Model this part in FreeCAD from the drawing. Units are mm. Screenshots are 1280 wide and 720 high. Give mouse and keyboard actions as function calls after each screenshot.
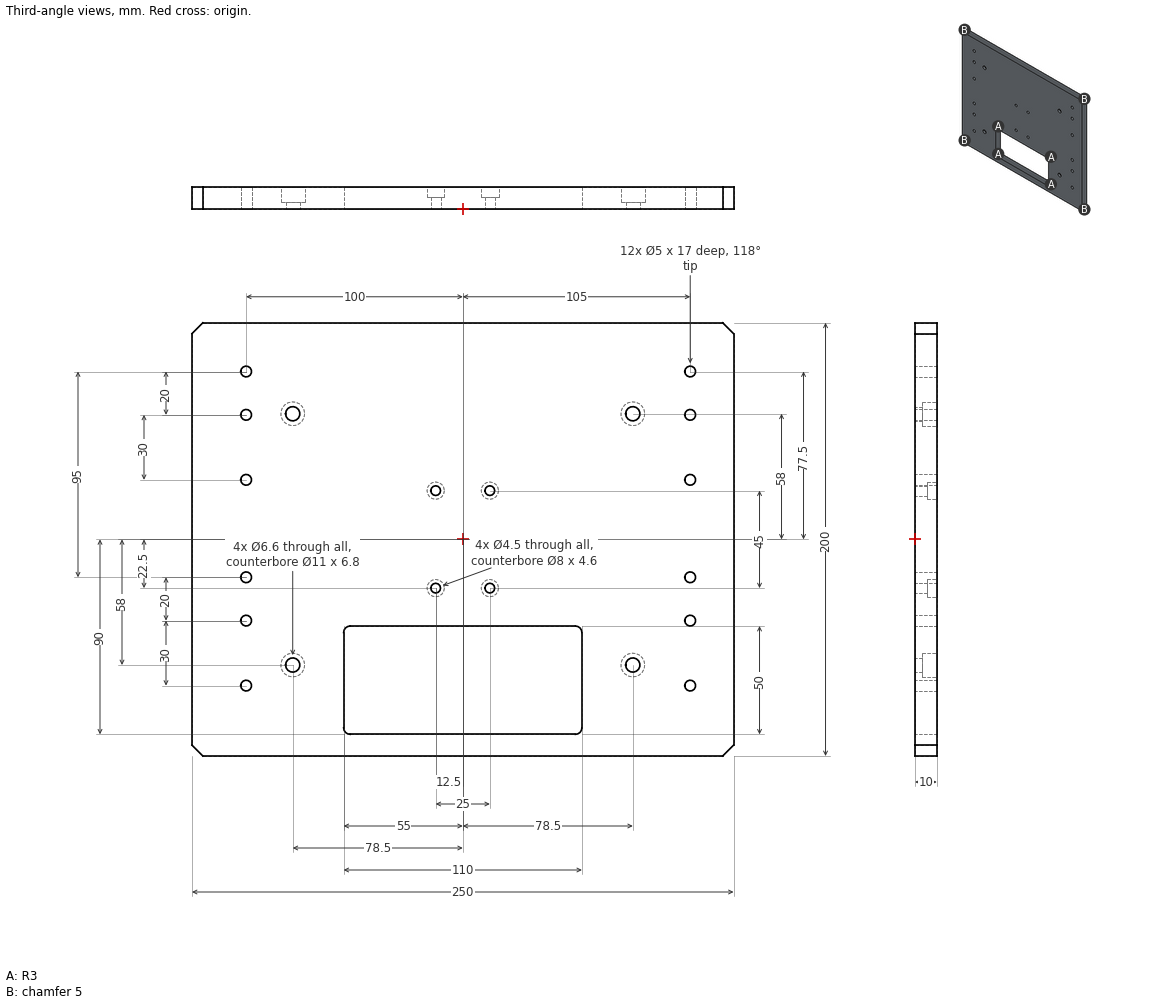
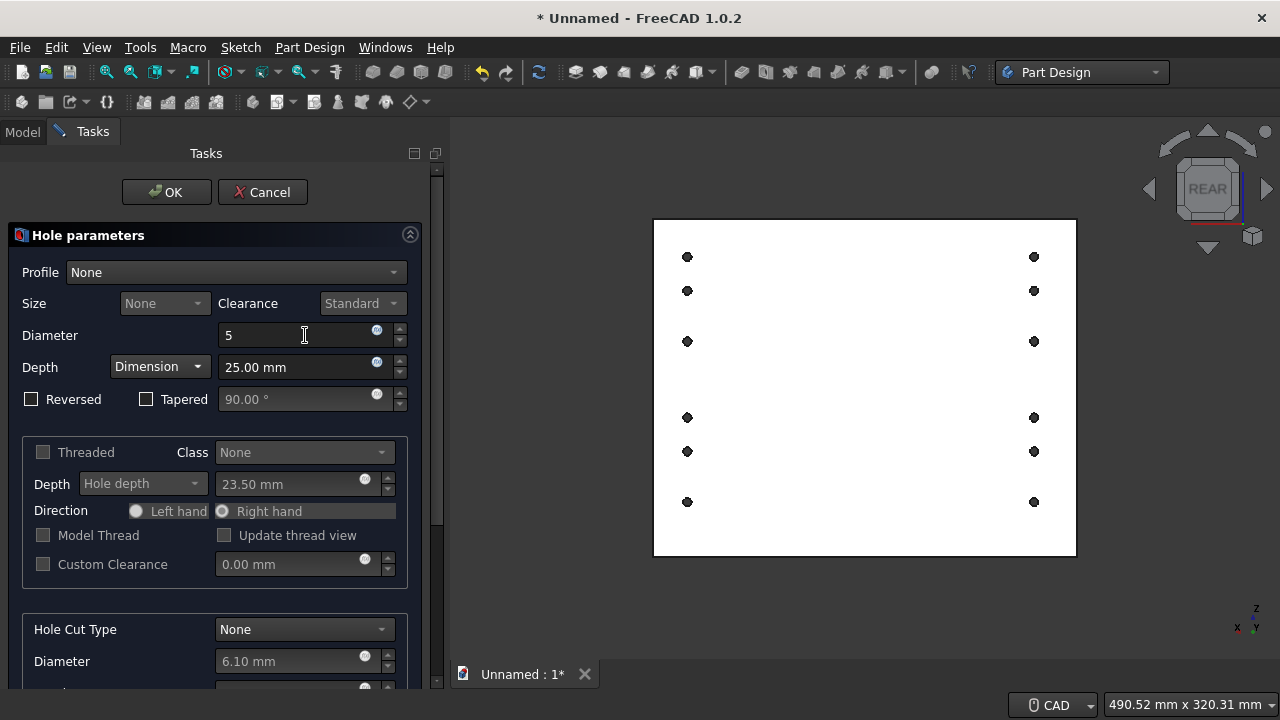
triple_click(305, 367)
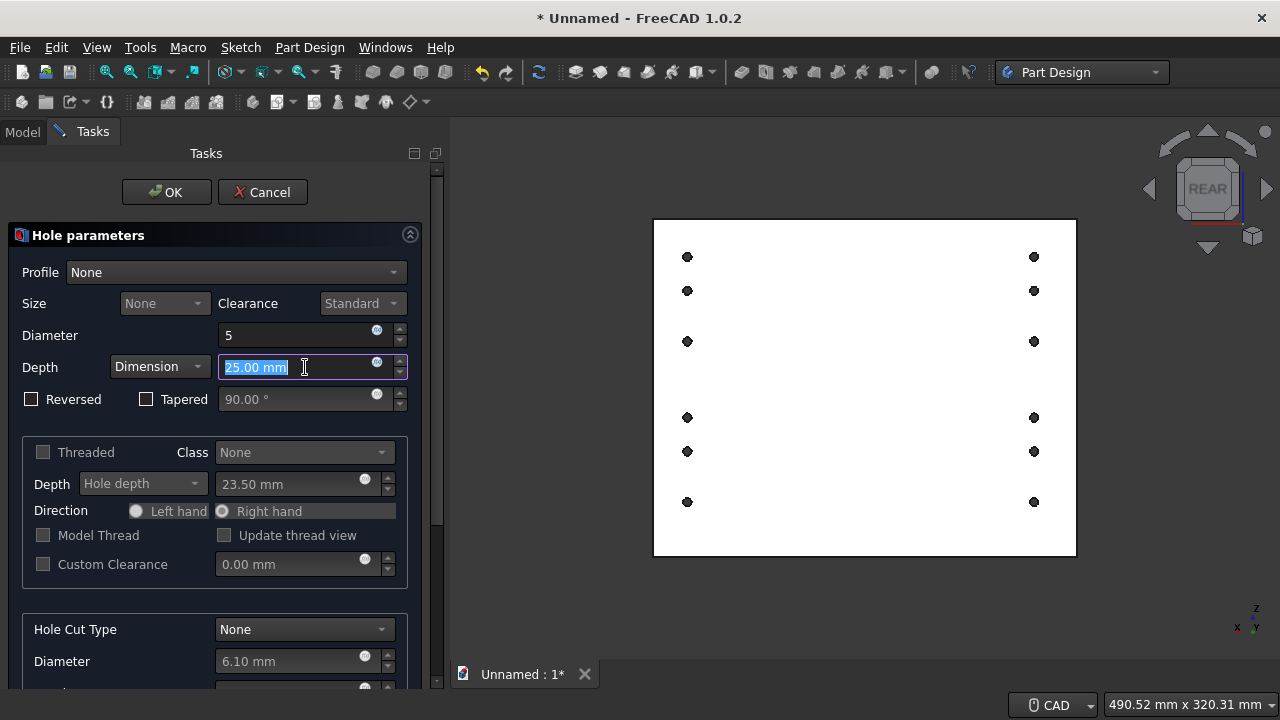
text(17)
key(Tab)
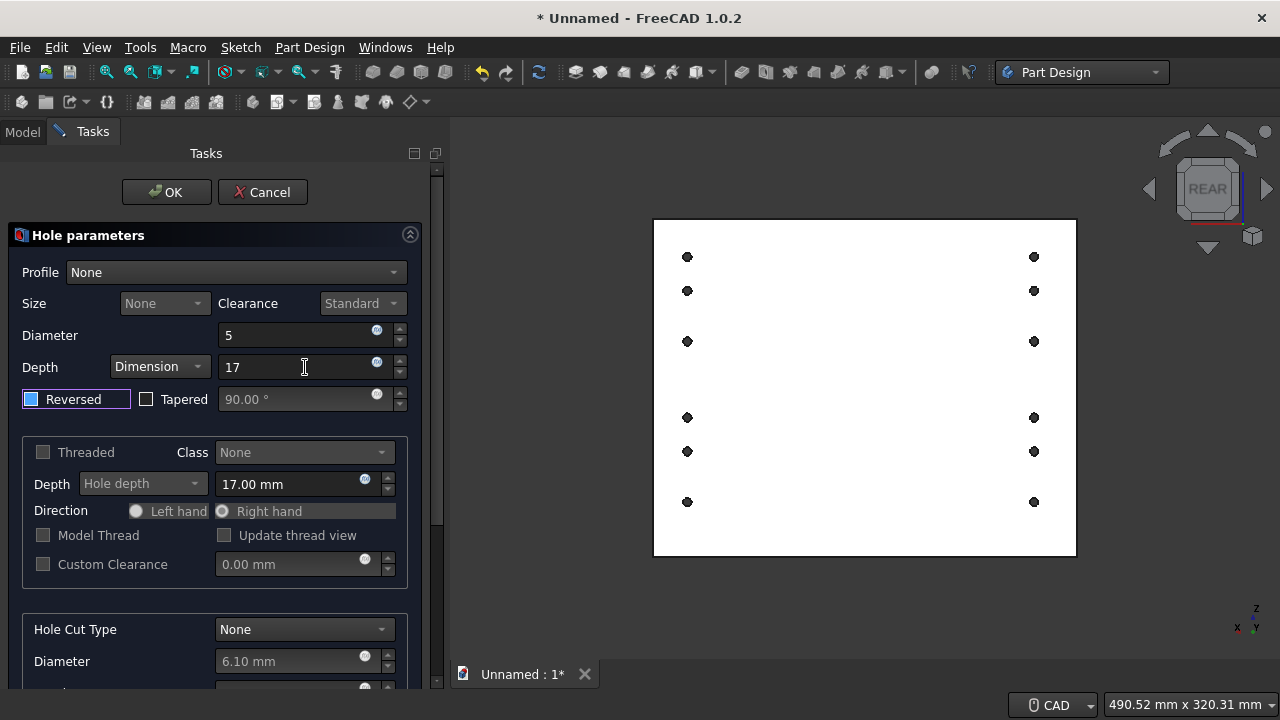
click(167, 192)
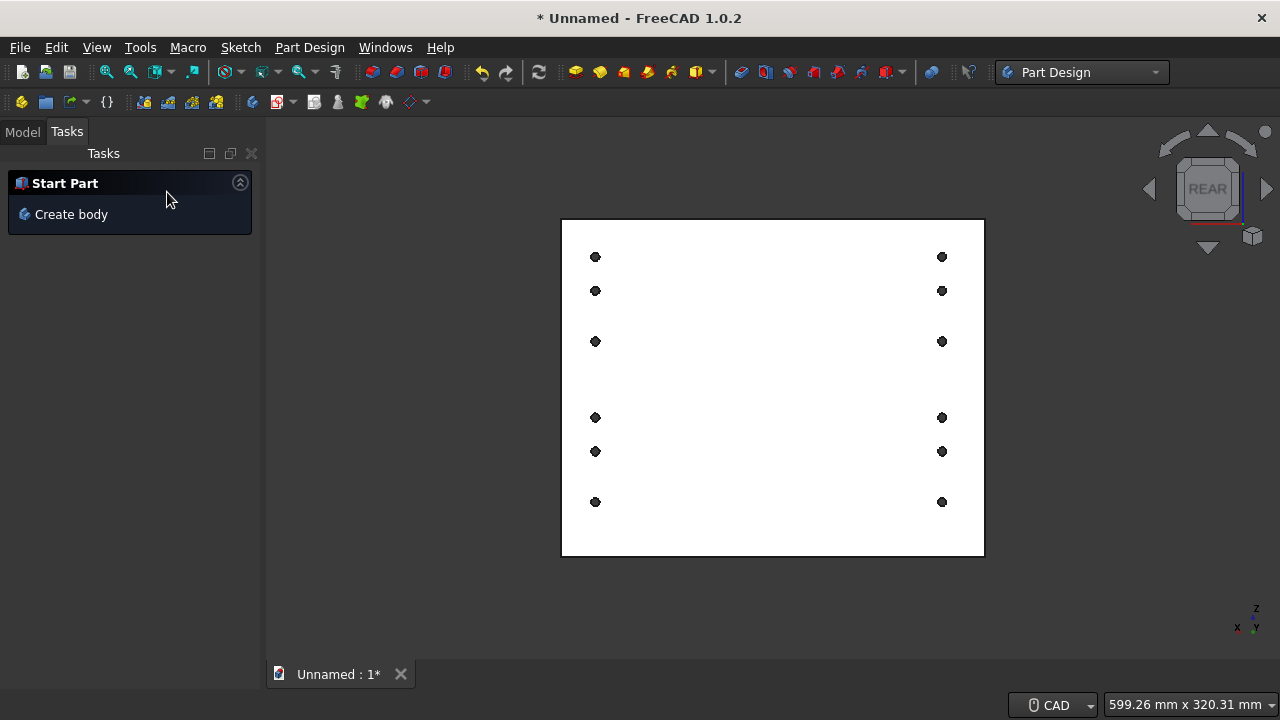
click(773, 387)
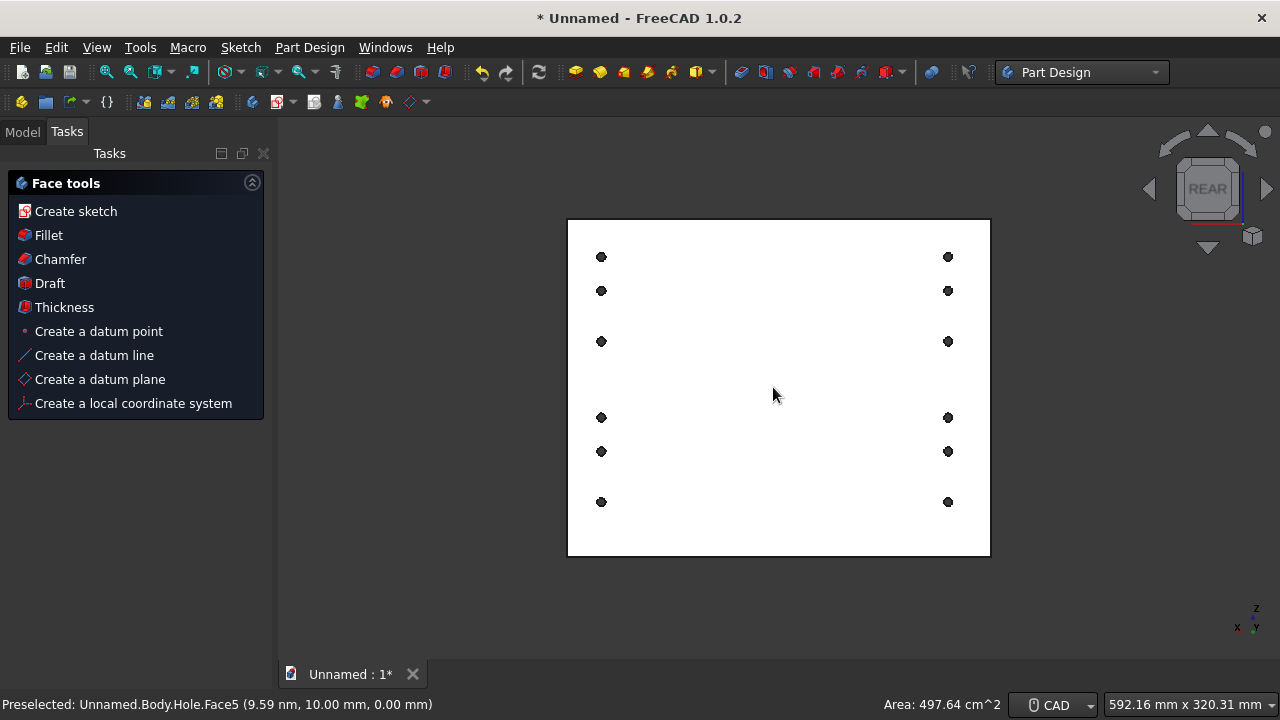
click(278, 102)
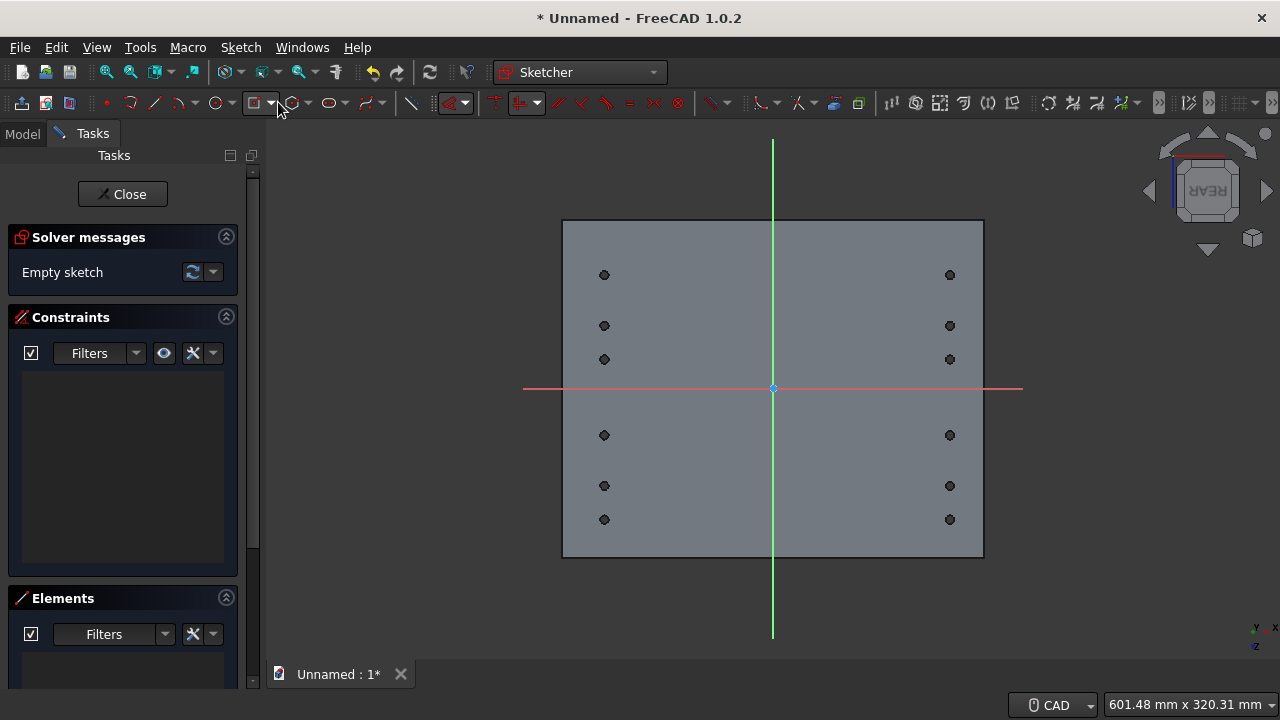
scroll(829, 251, up, 4)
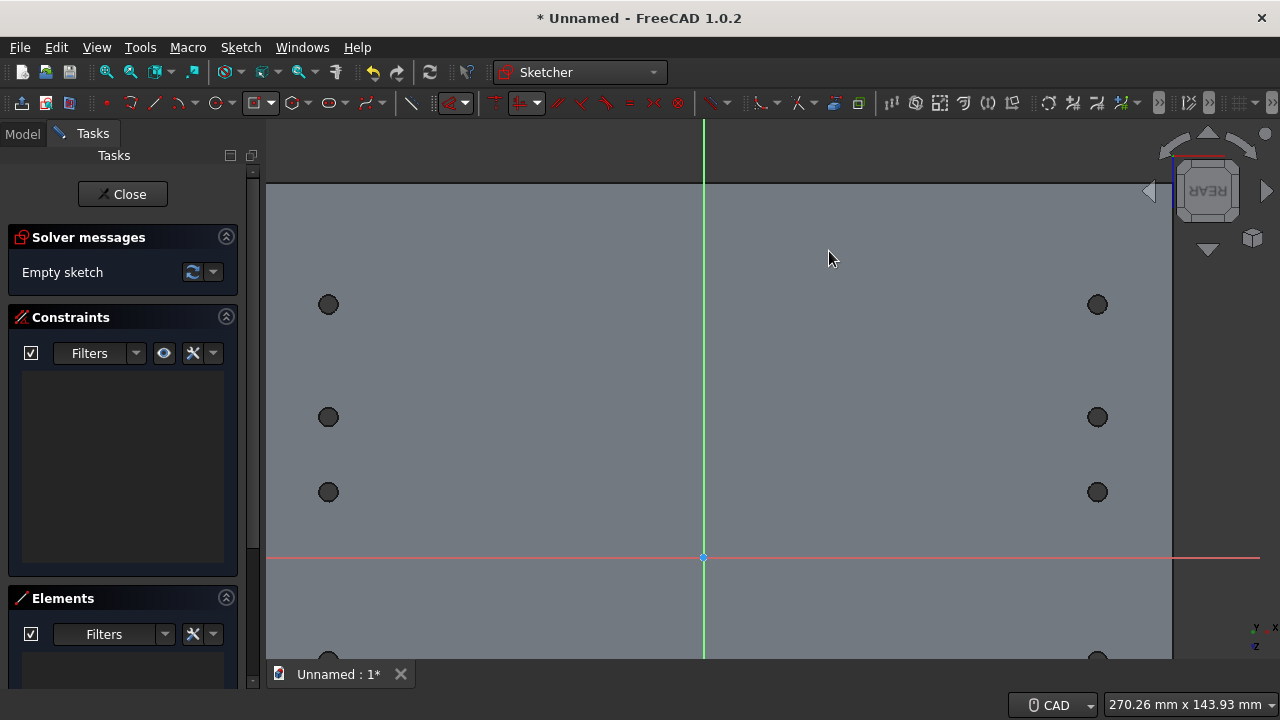
key(g)
key(r)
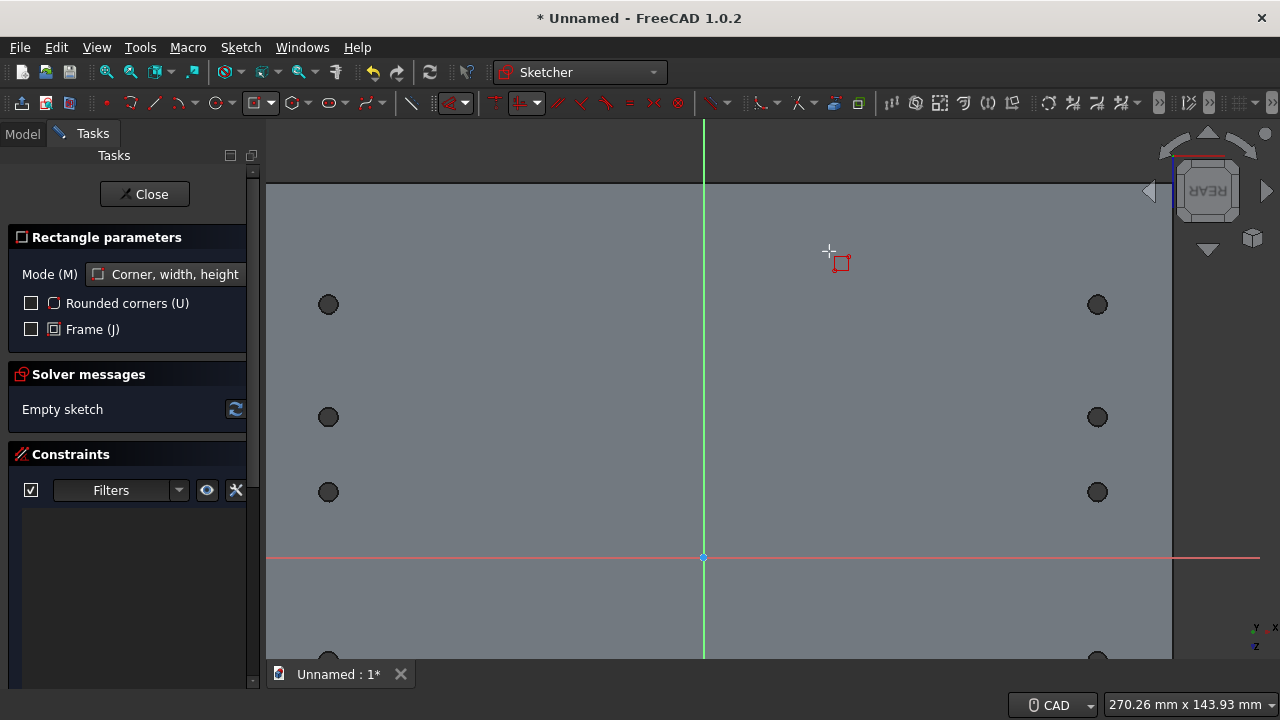
click(497, 220)
move(910, 408)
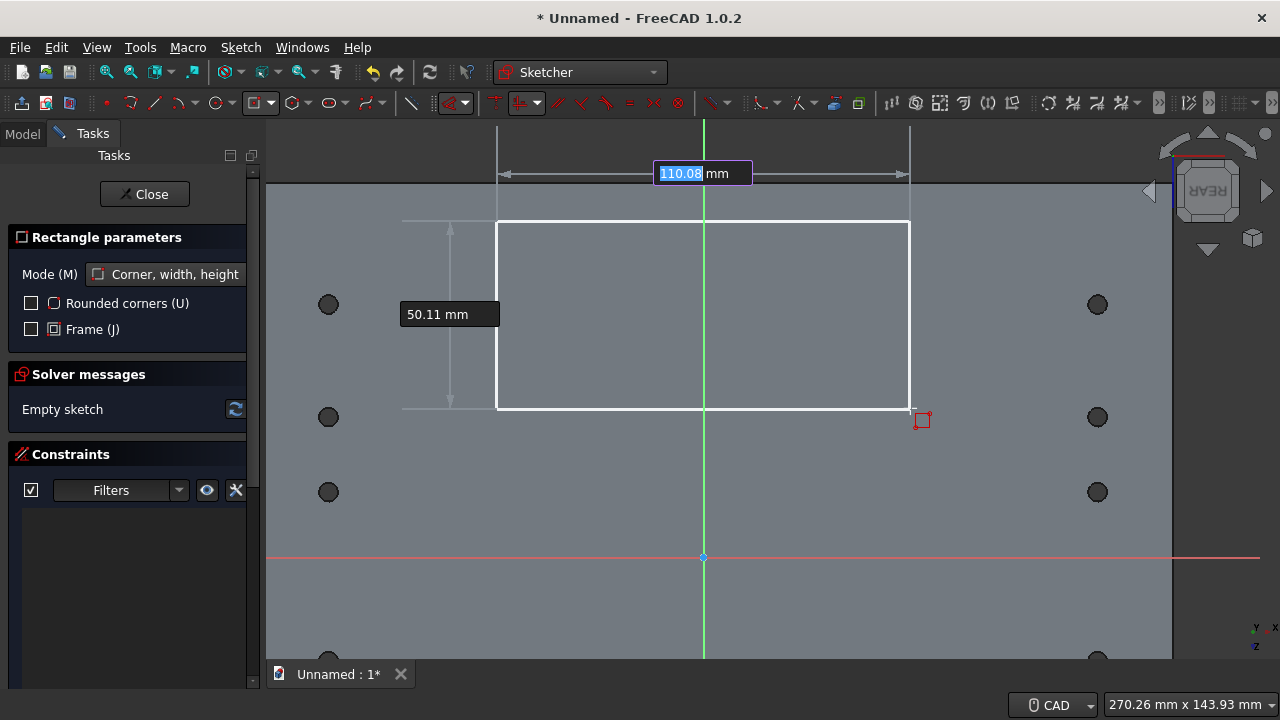
text(110)
key(Tab)
text(50)
key(Return)
key(Escape)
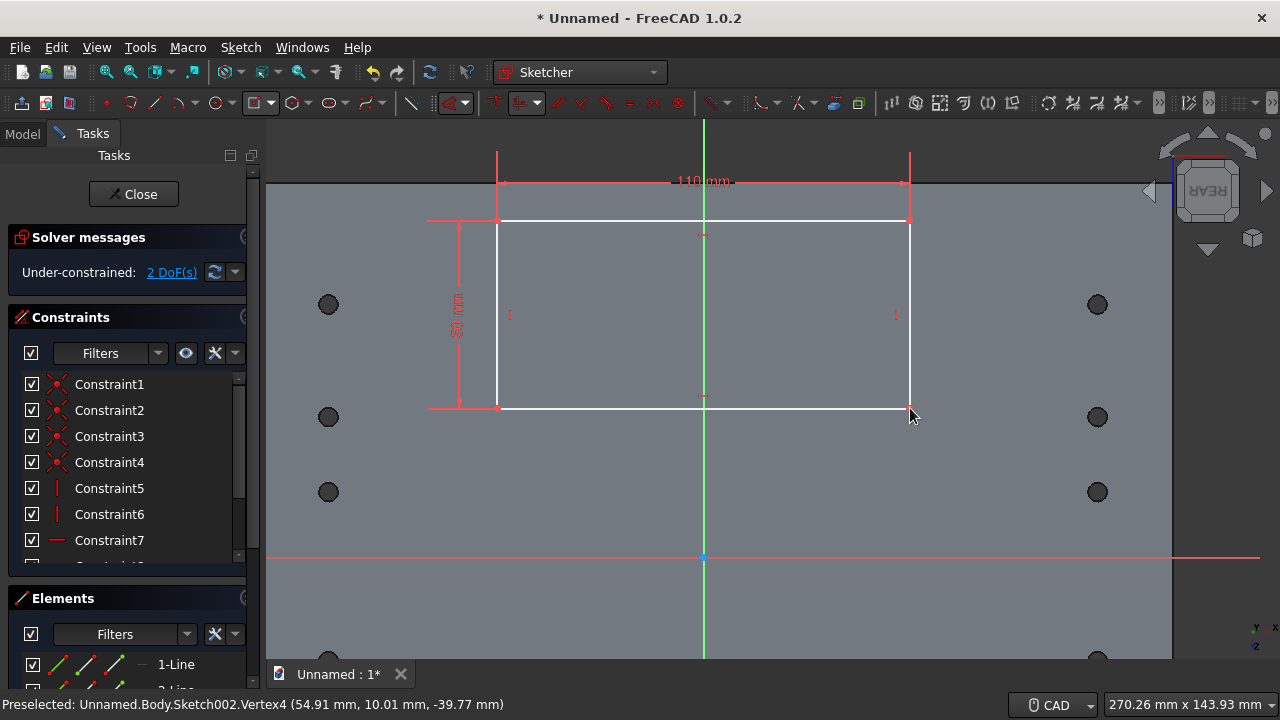
click(497, 221)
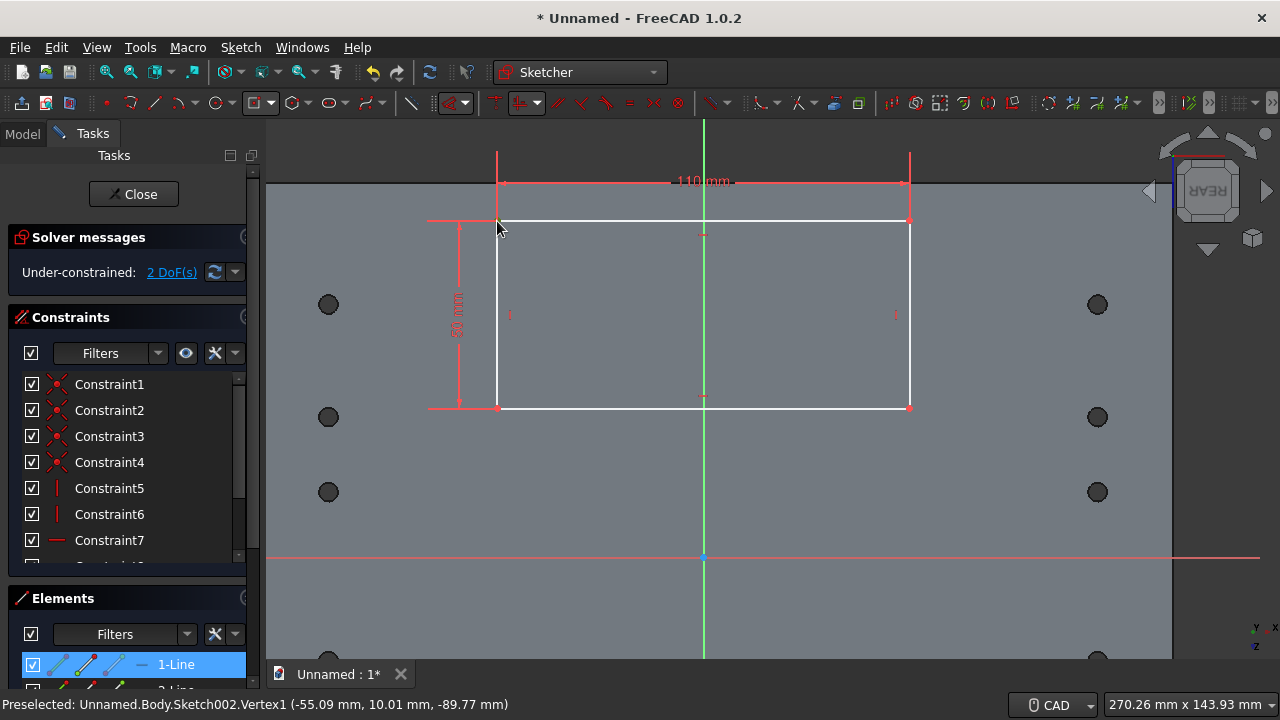
key(l)